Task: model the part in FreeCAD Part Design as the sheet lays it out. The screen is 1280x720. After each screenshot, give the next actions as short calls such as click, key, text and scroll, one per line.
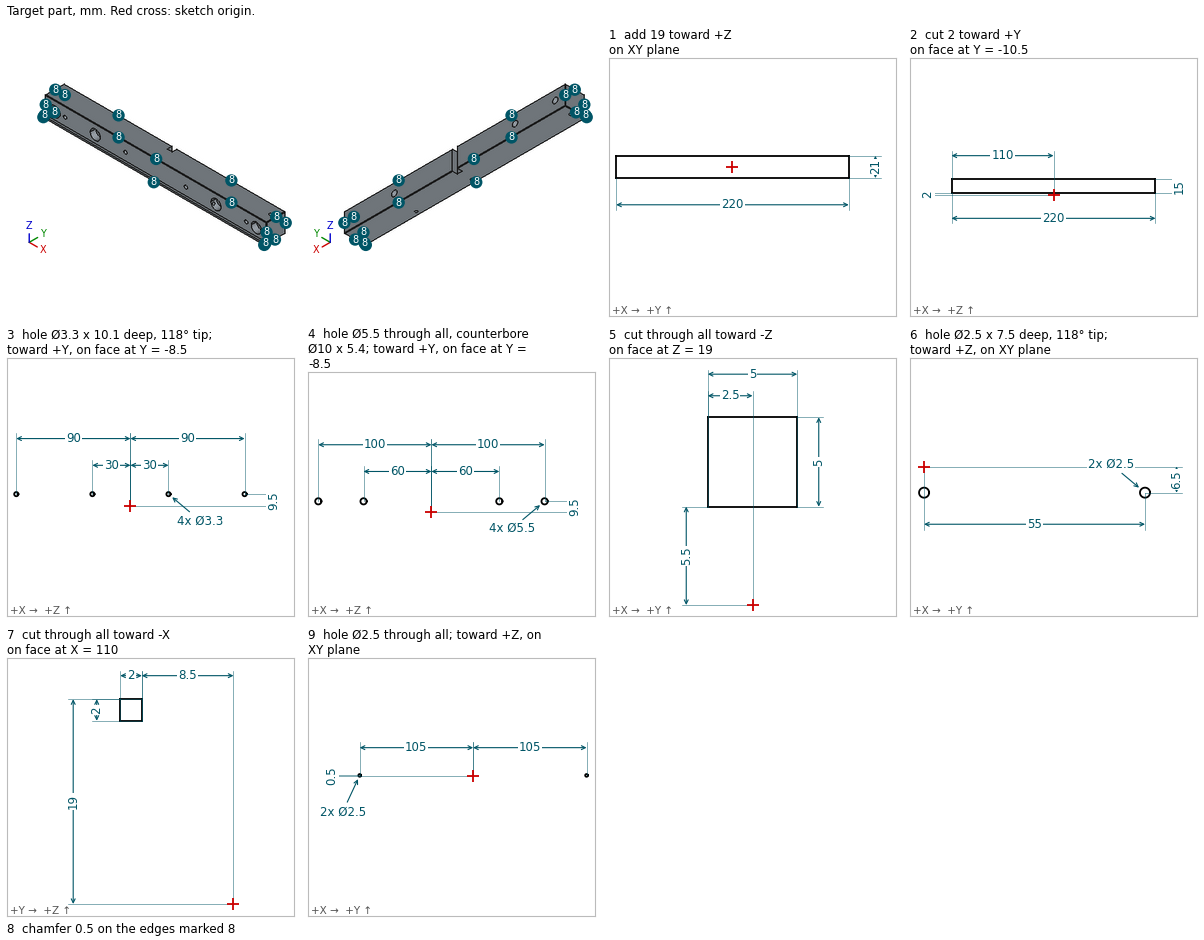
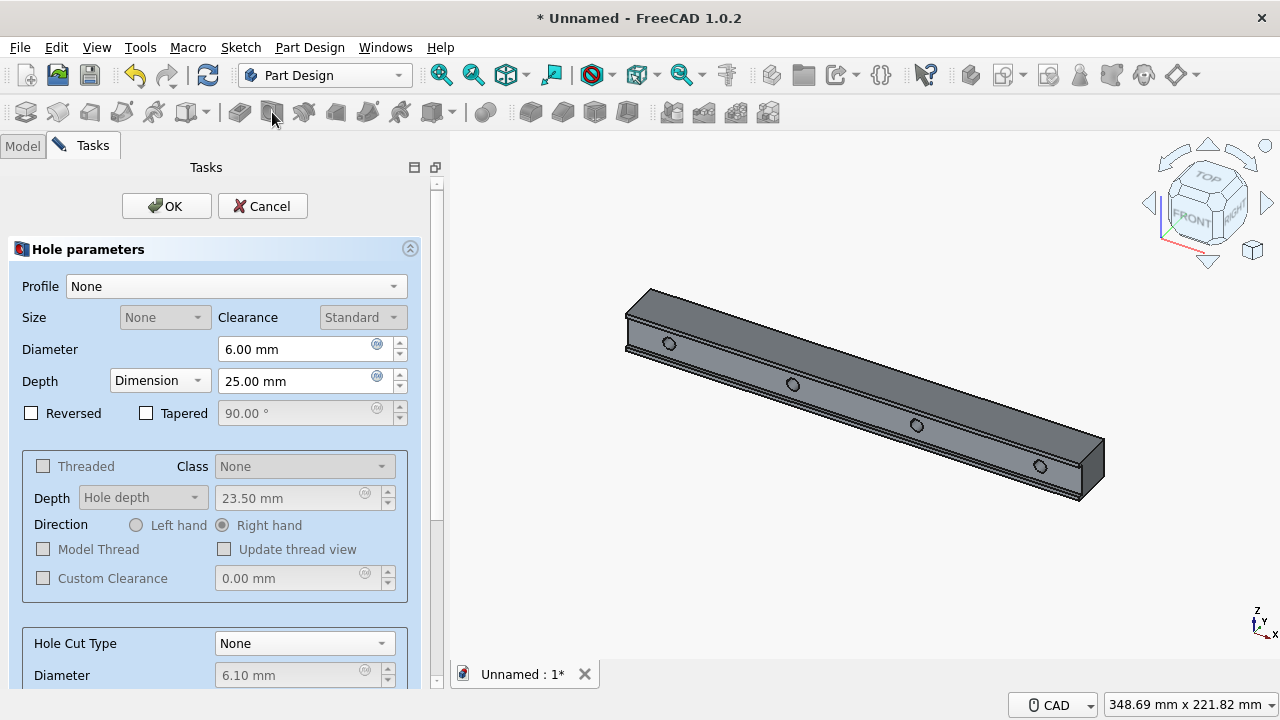
triple_click(305, 349)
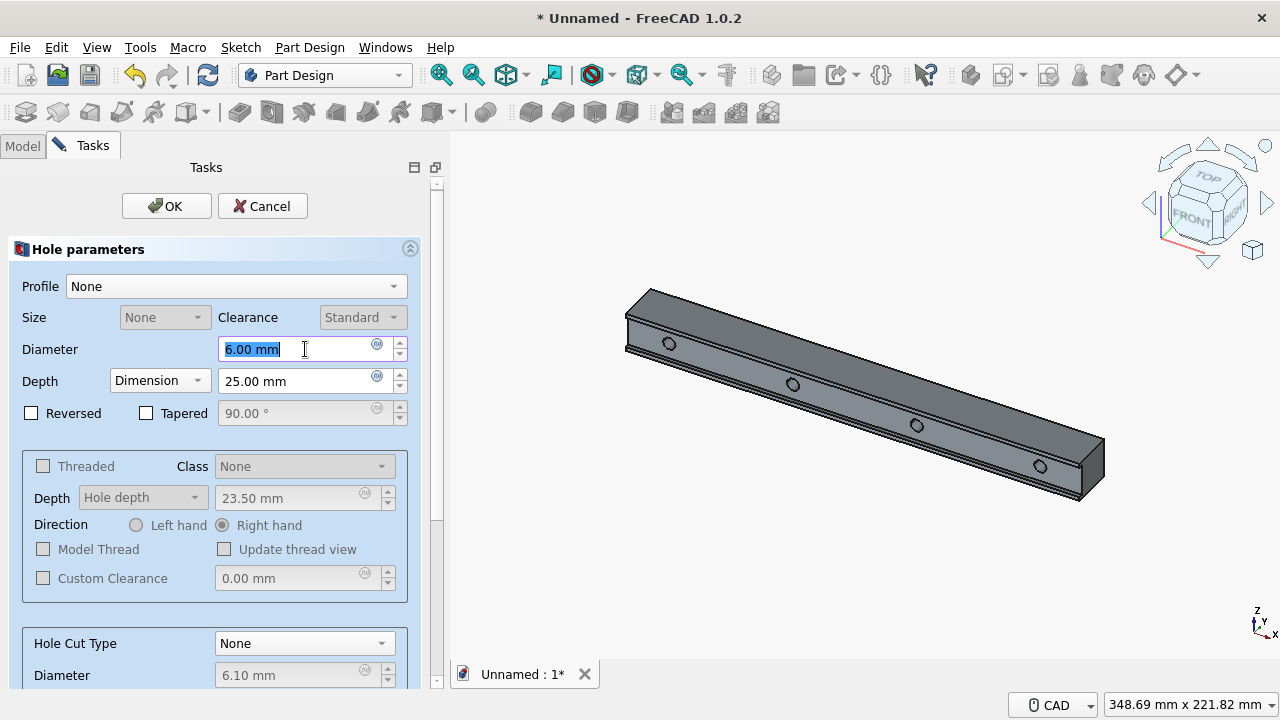
text(3.3)
key(Tab)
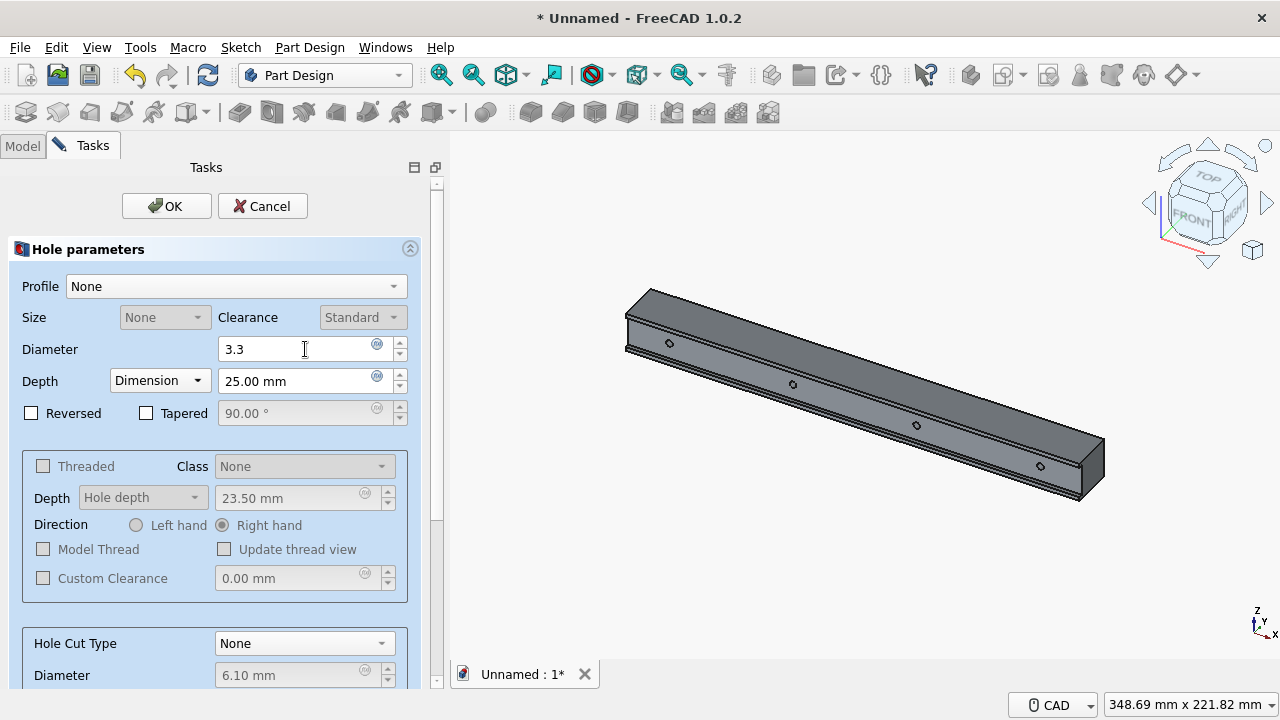
triple_click(305, 381)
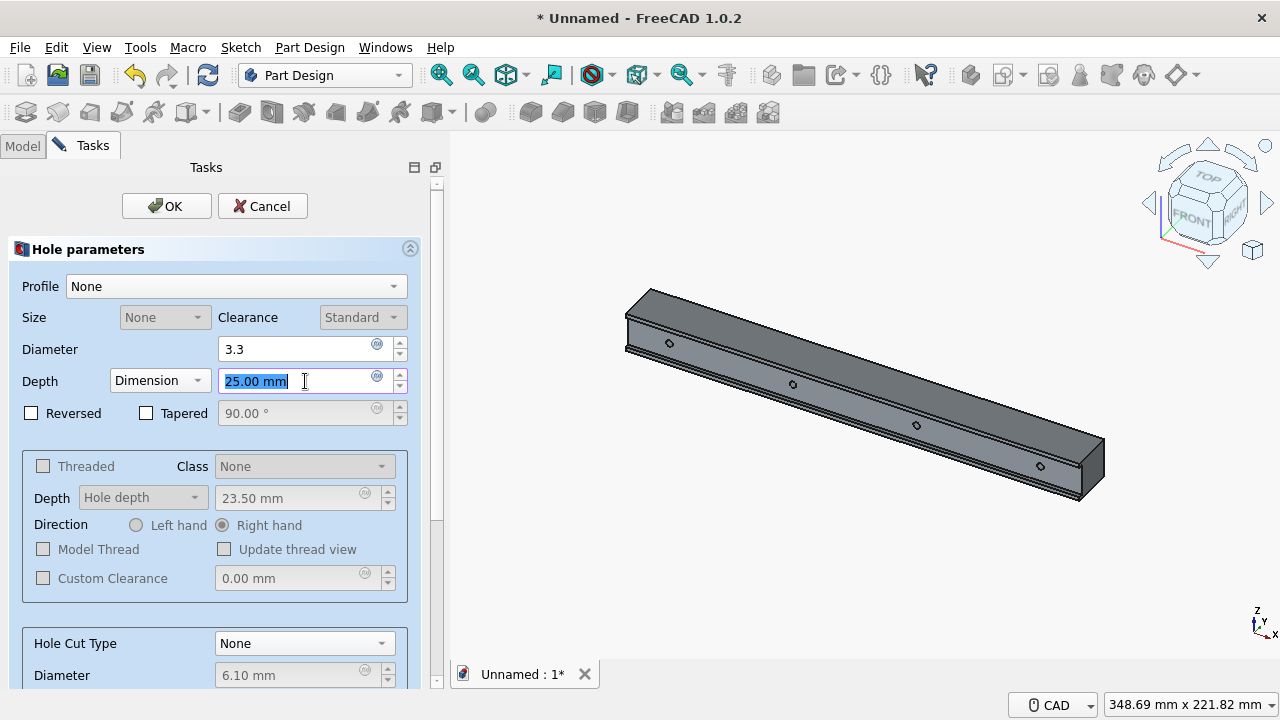
text(10.1)
key(Tab)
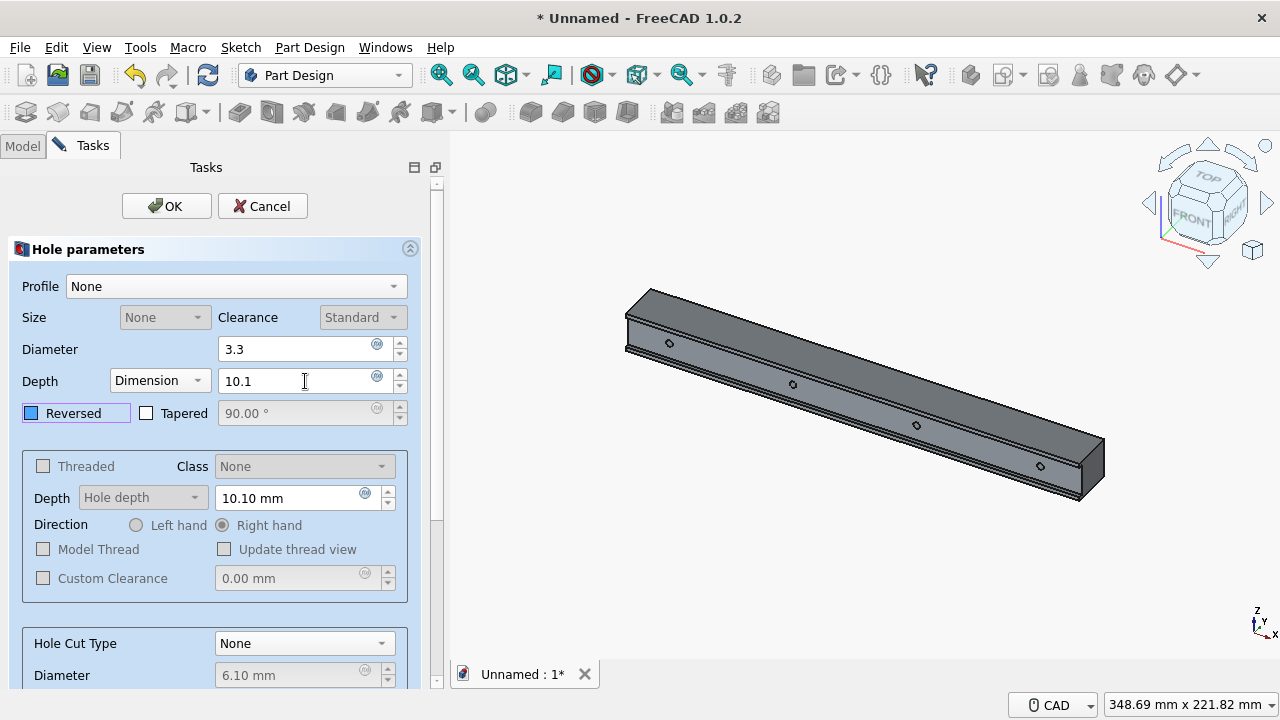
click(167, 206)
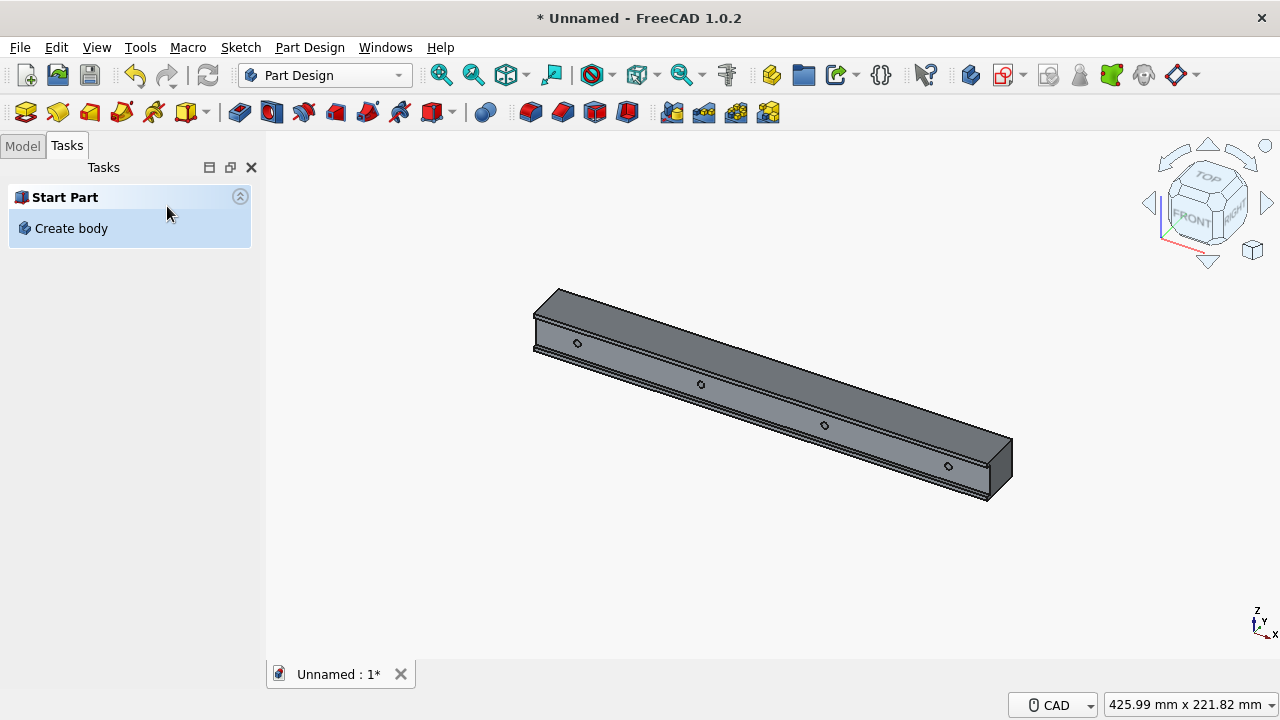
click(892, 447)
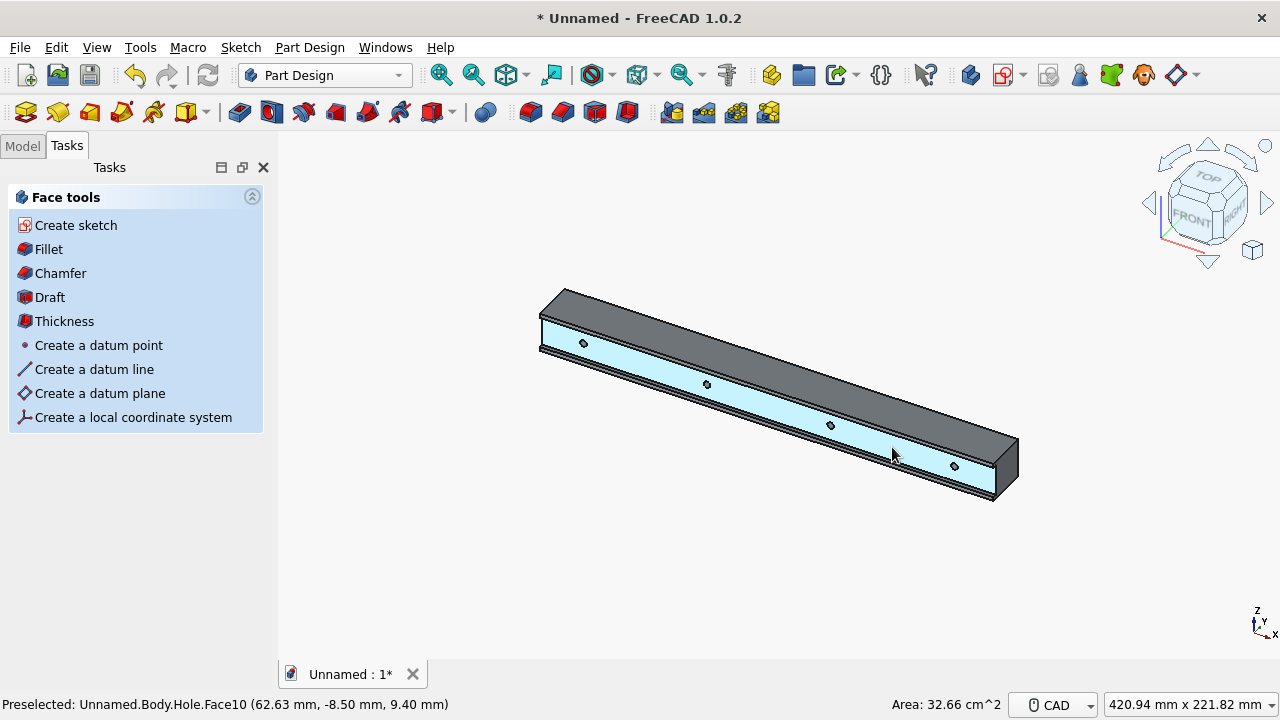
click(1004, 76)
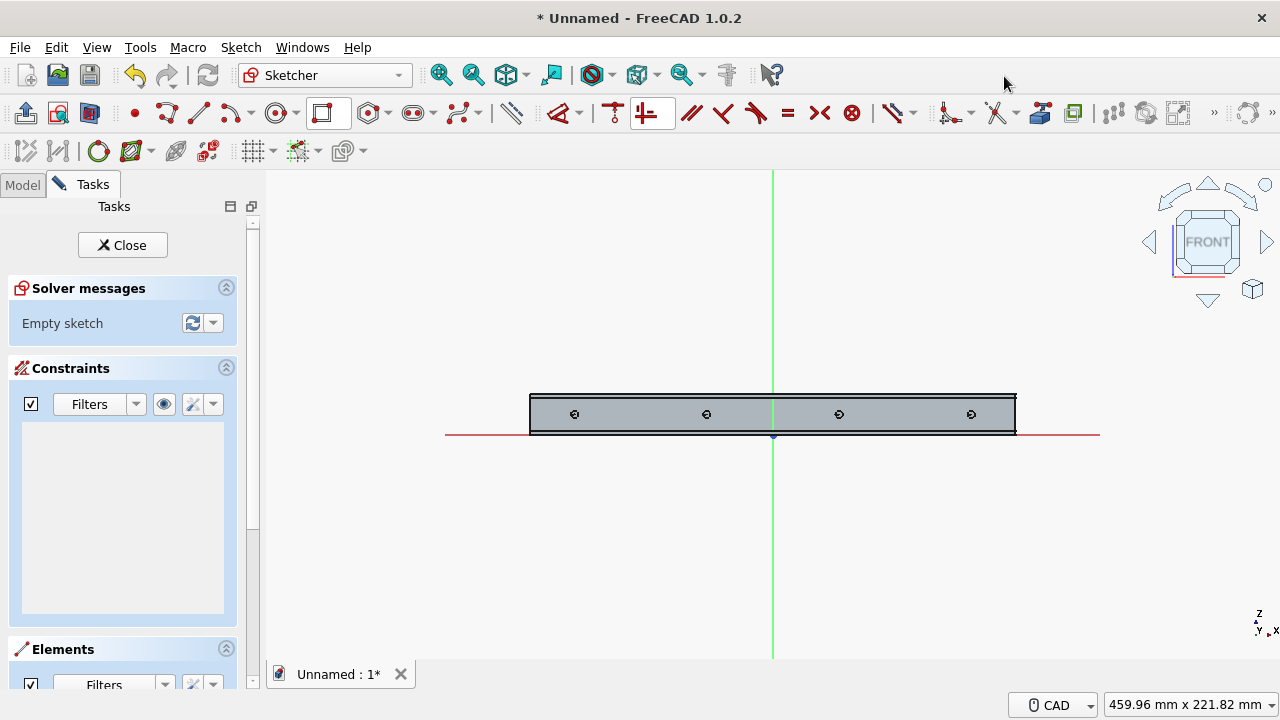
click(276, 114)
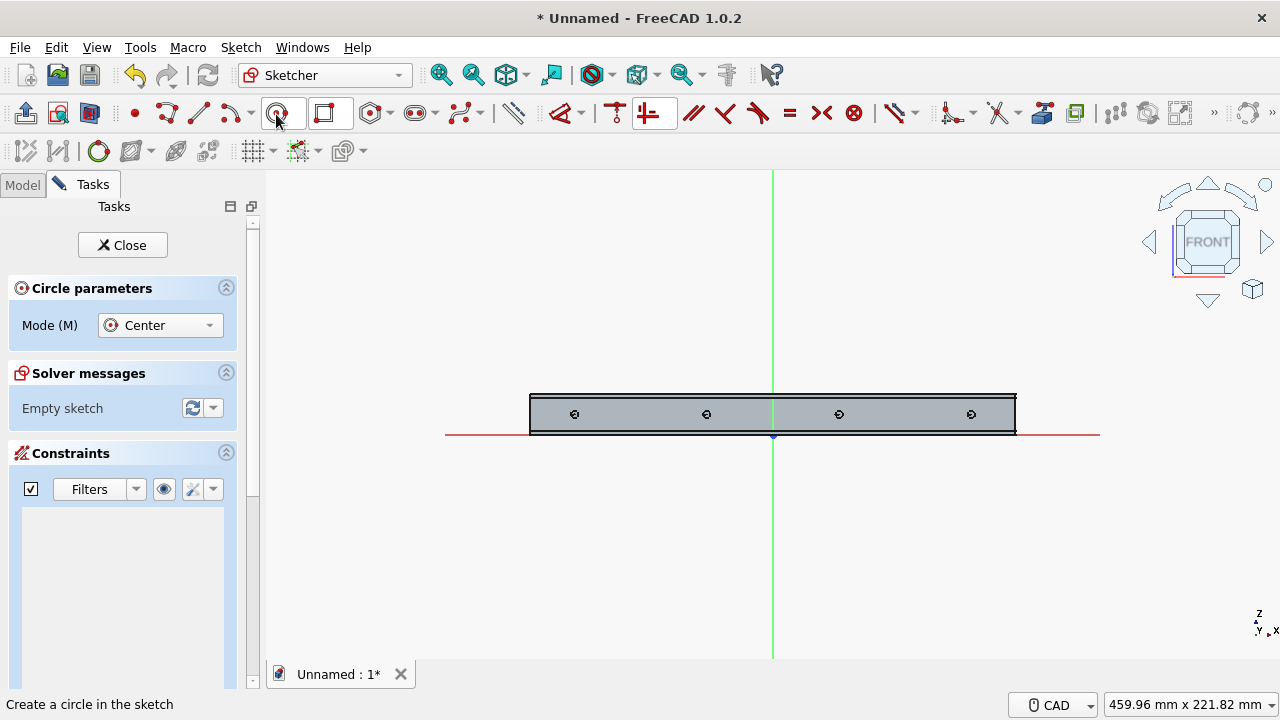
scroll(993, 415, up, 7)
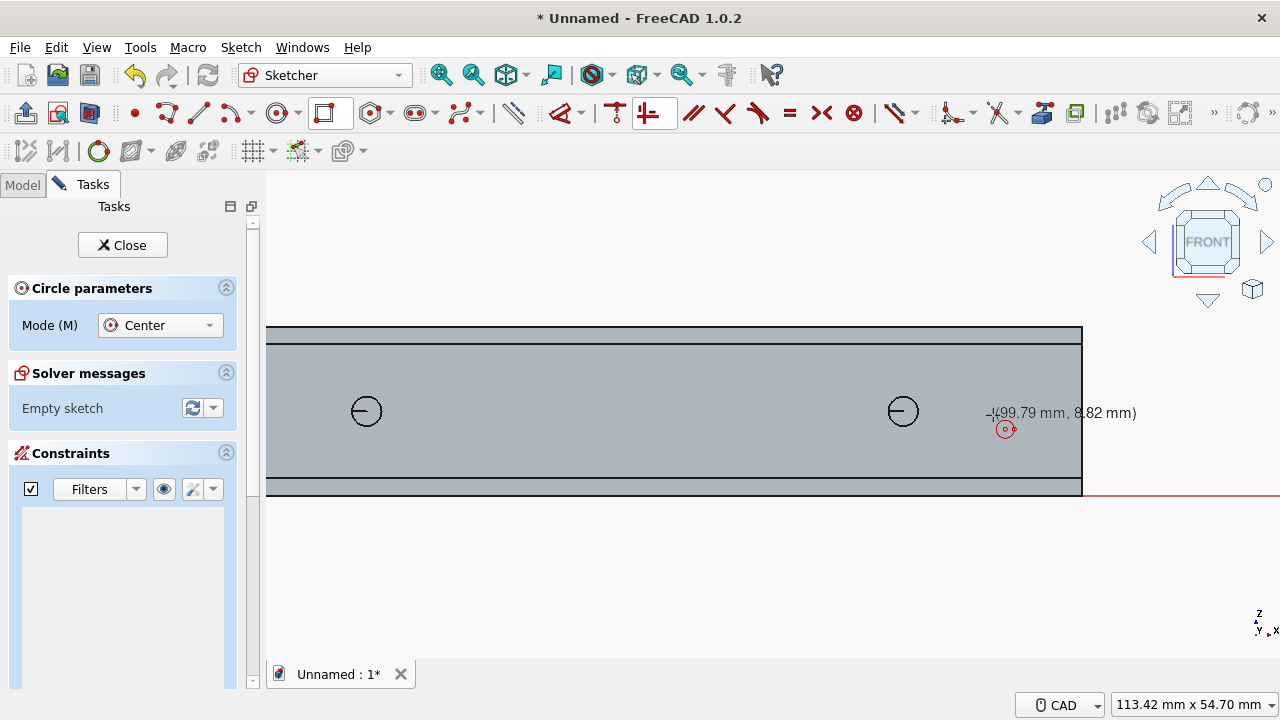
scroll(966, 403, down, 6)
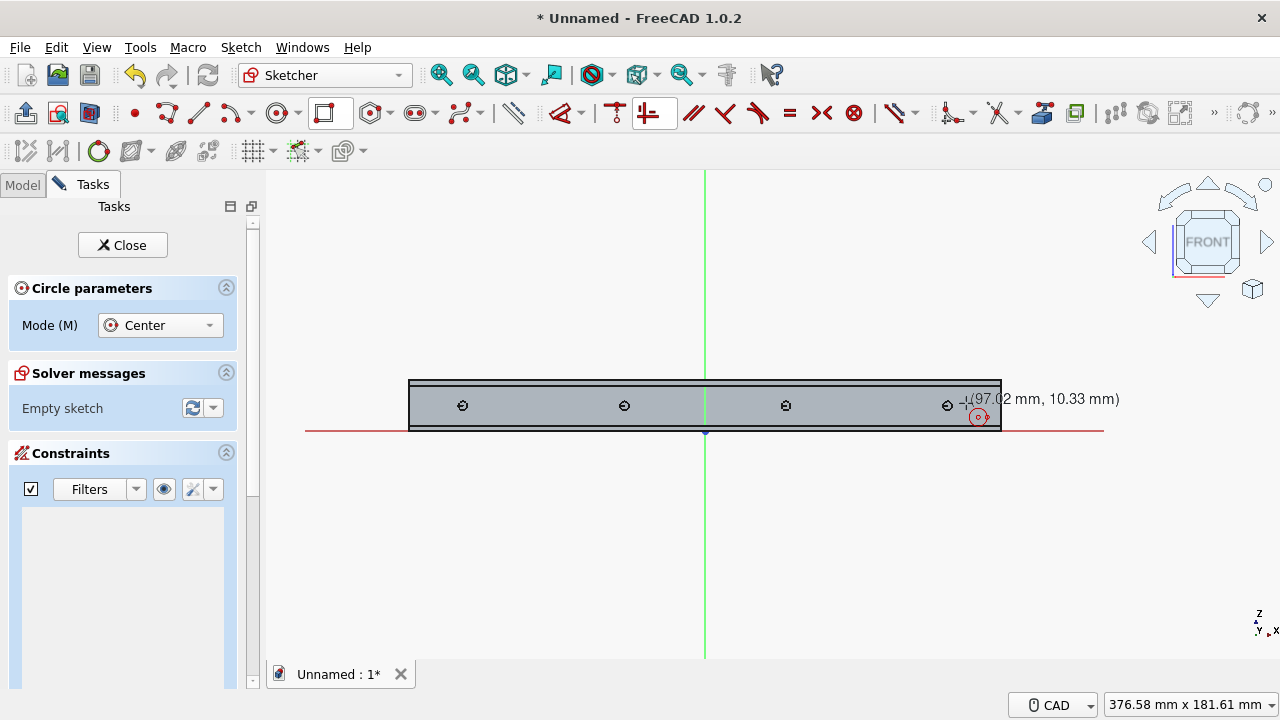
click(975, 406)
move(980, 401)